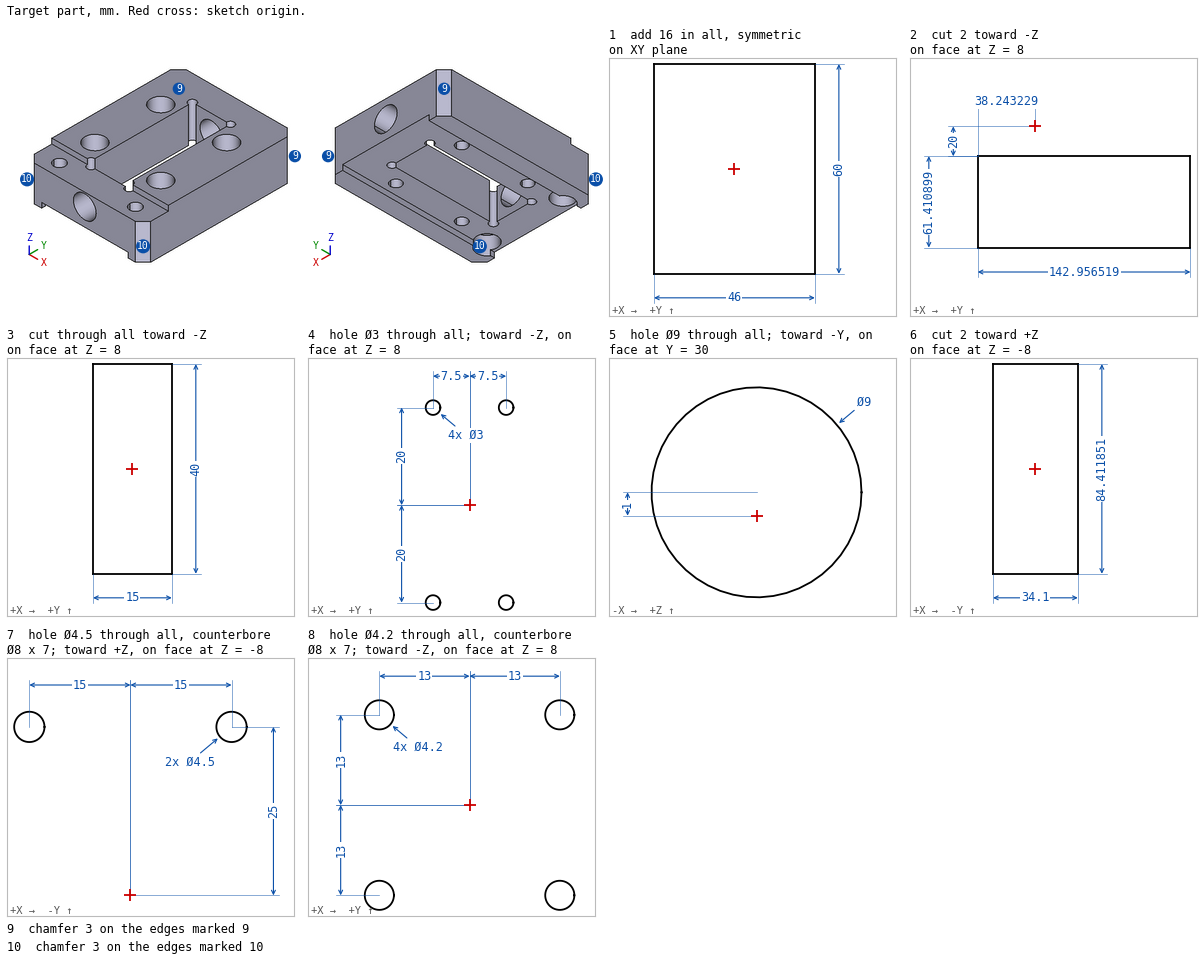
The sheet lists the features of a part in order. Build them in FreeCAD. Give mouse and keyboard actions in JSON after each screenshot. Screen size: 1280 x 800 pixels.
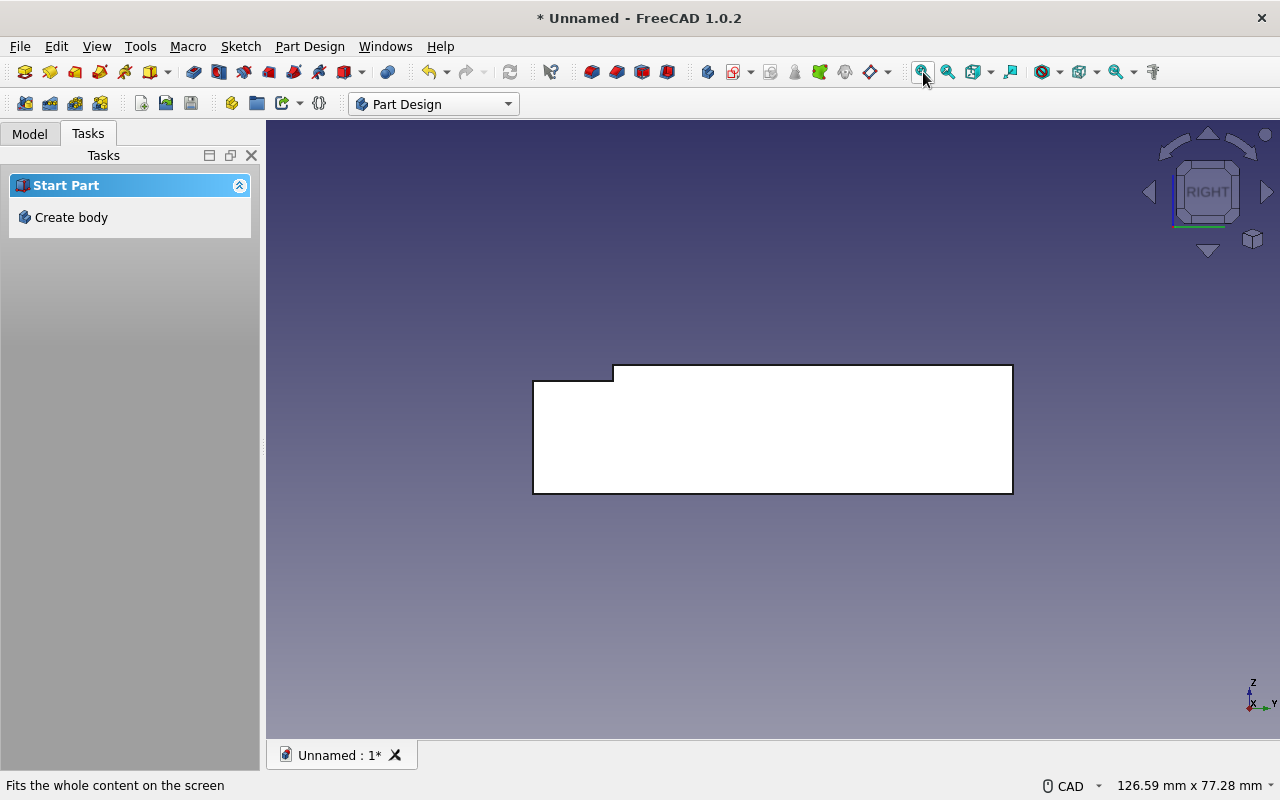
{"action": "left_click", "coordinate": [1013, 428]}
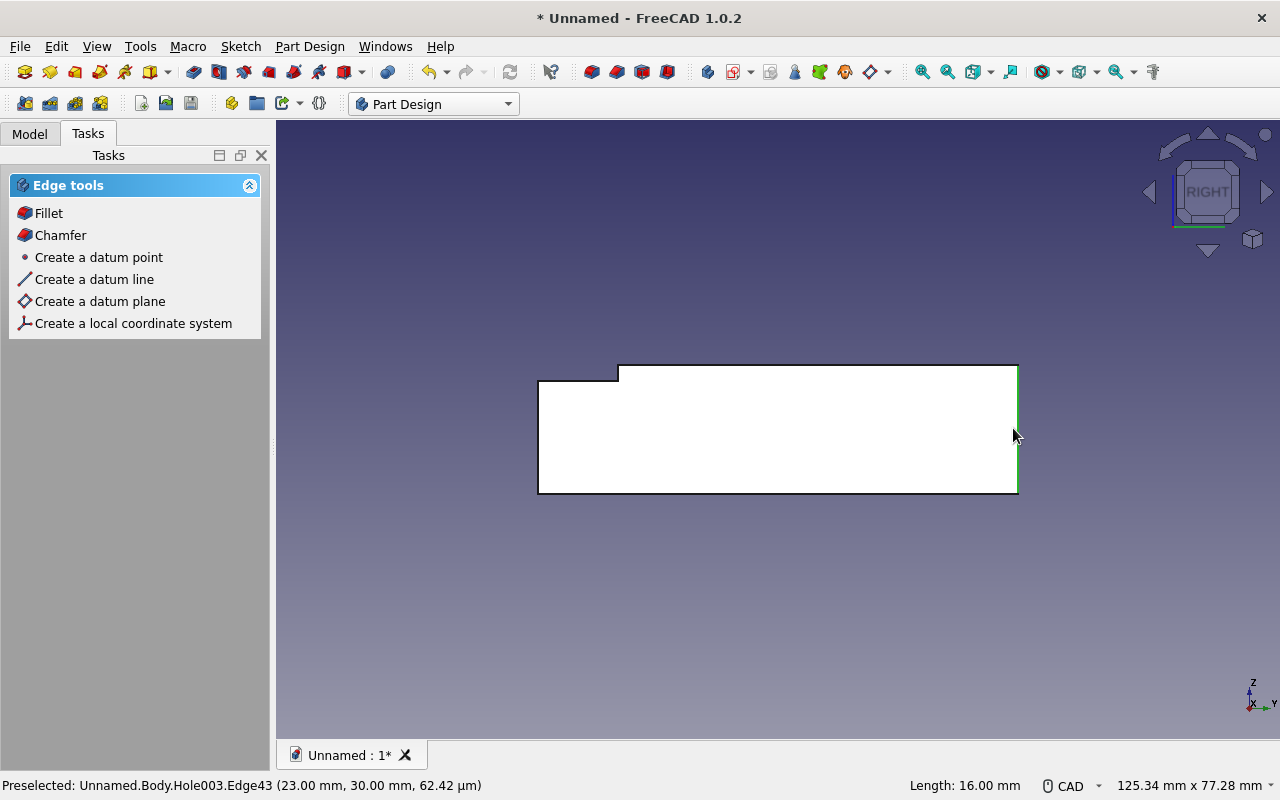
{"action": "key", "text": "5"}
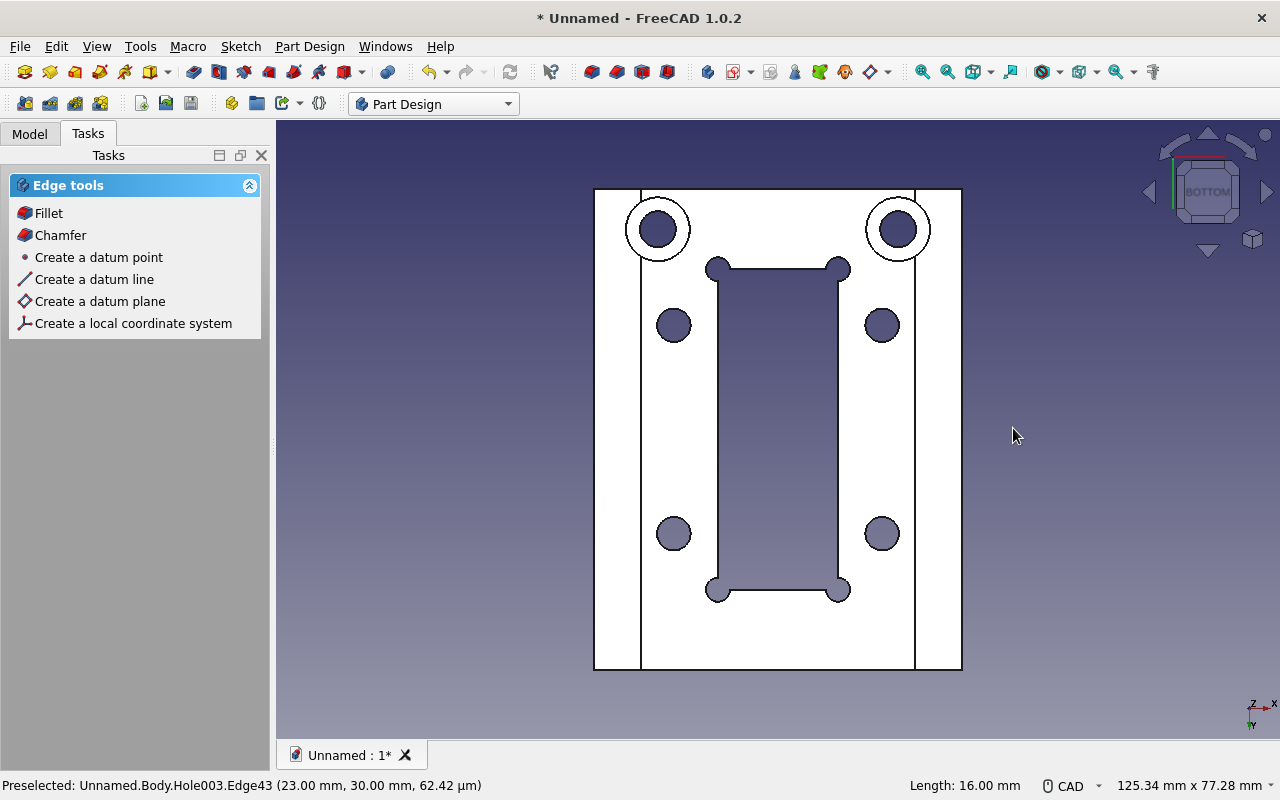
{"action": "key", "text": "4"}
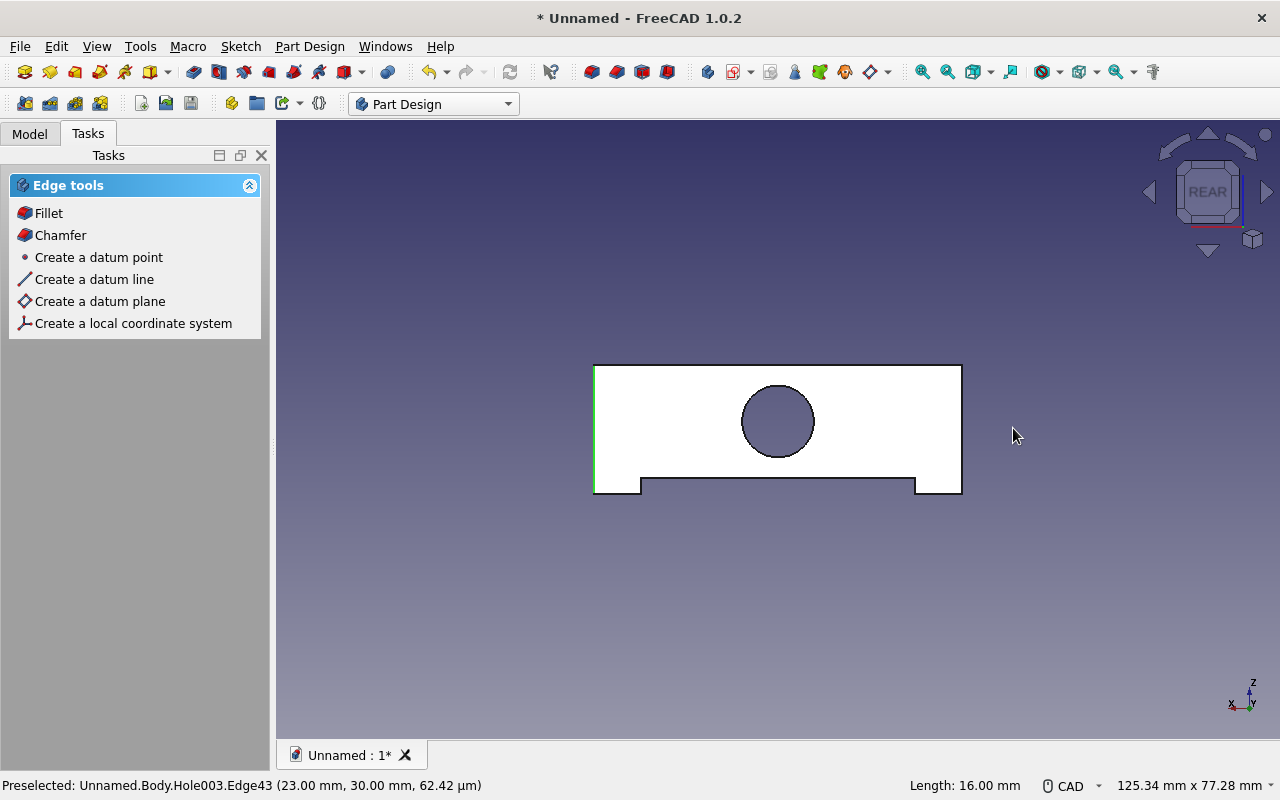
{"action": "left_click", "coordinate": [923, 72]}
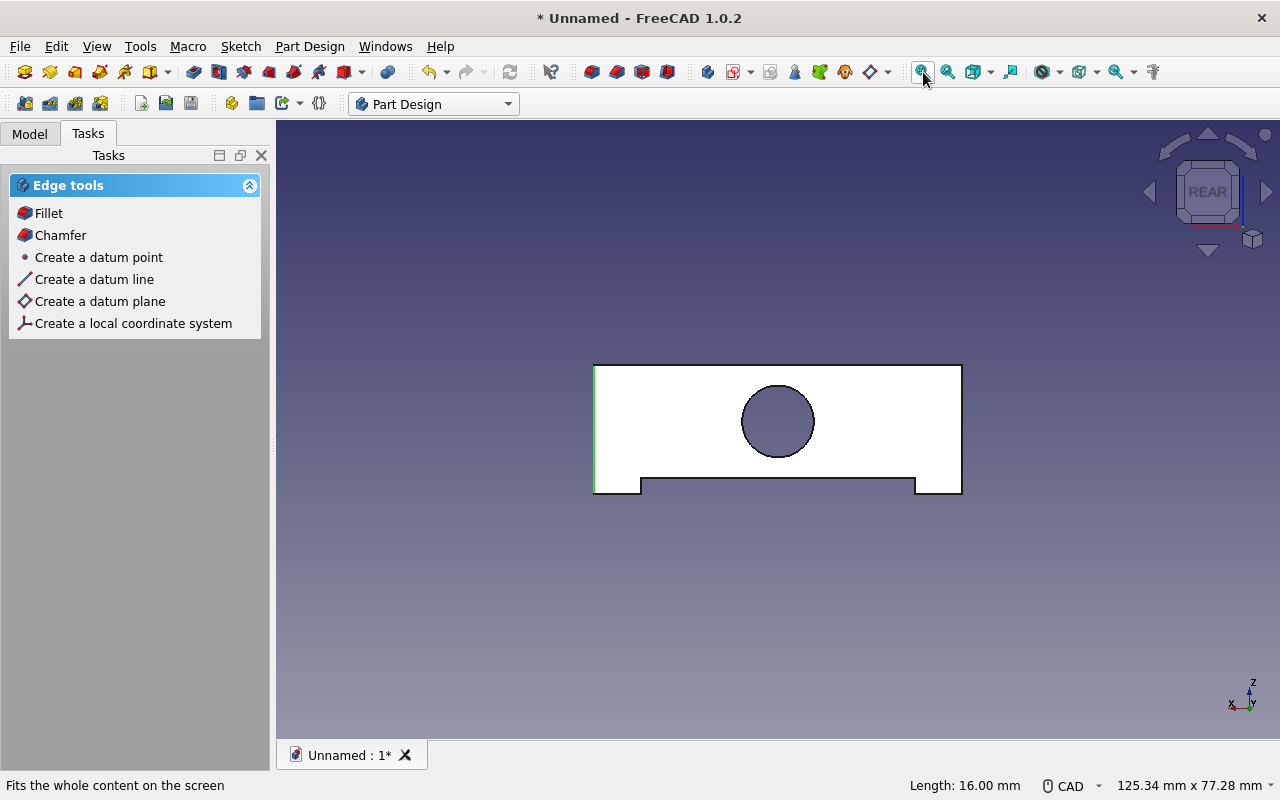
{"action": "left_click", "coordinate": [962, 429], "text": "ctrl"}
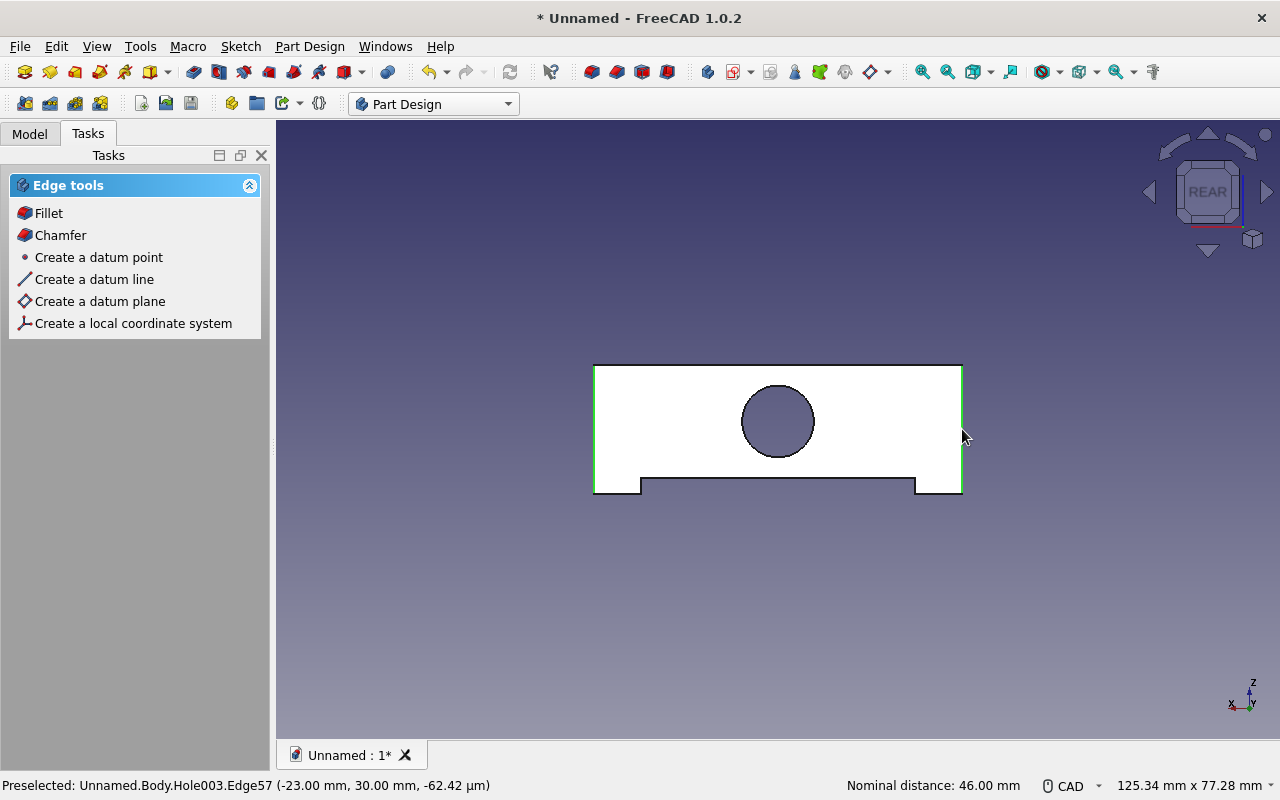
{"action": "left_click", "coordinate": [617, 72]}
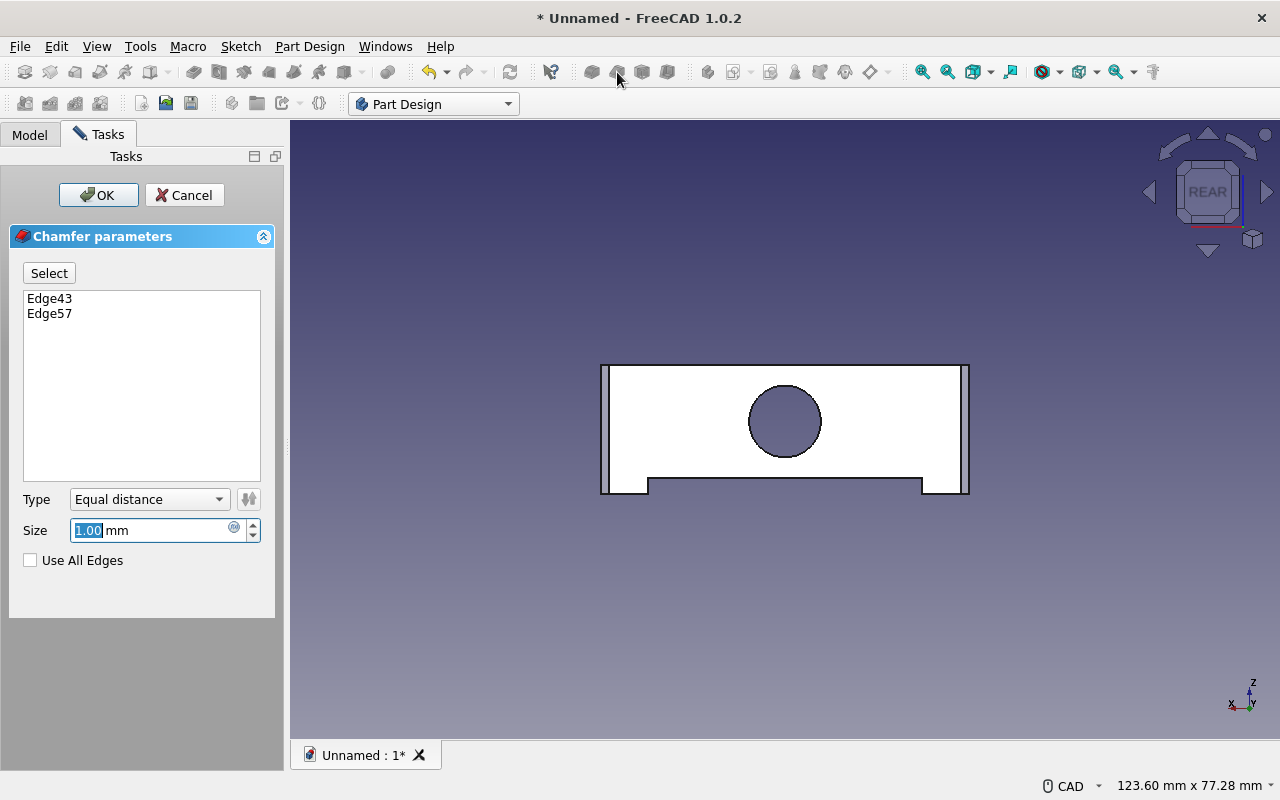
{"action": "type", "text": "3"}
{"action": "key", "text": "Tab"}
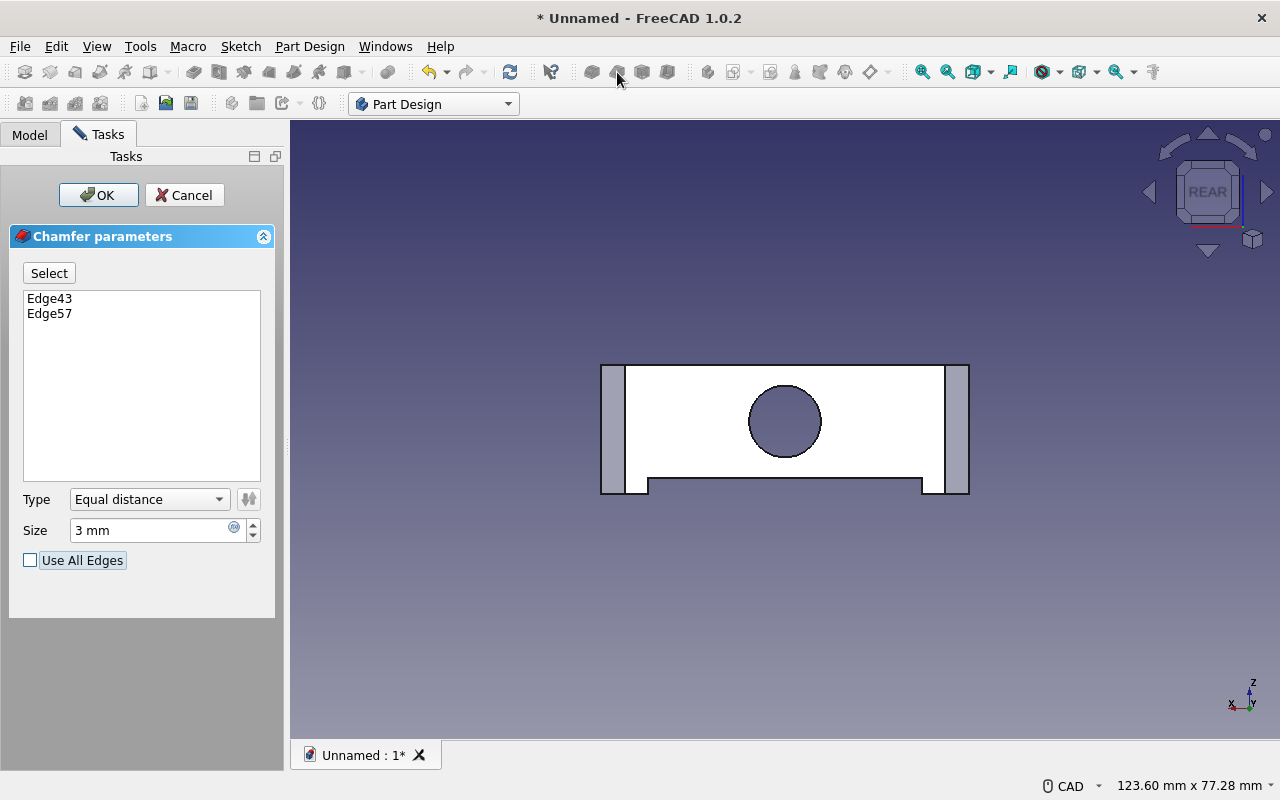
{"action": "left_click", "coordinate": [99, 195]}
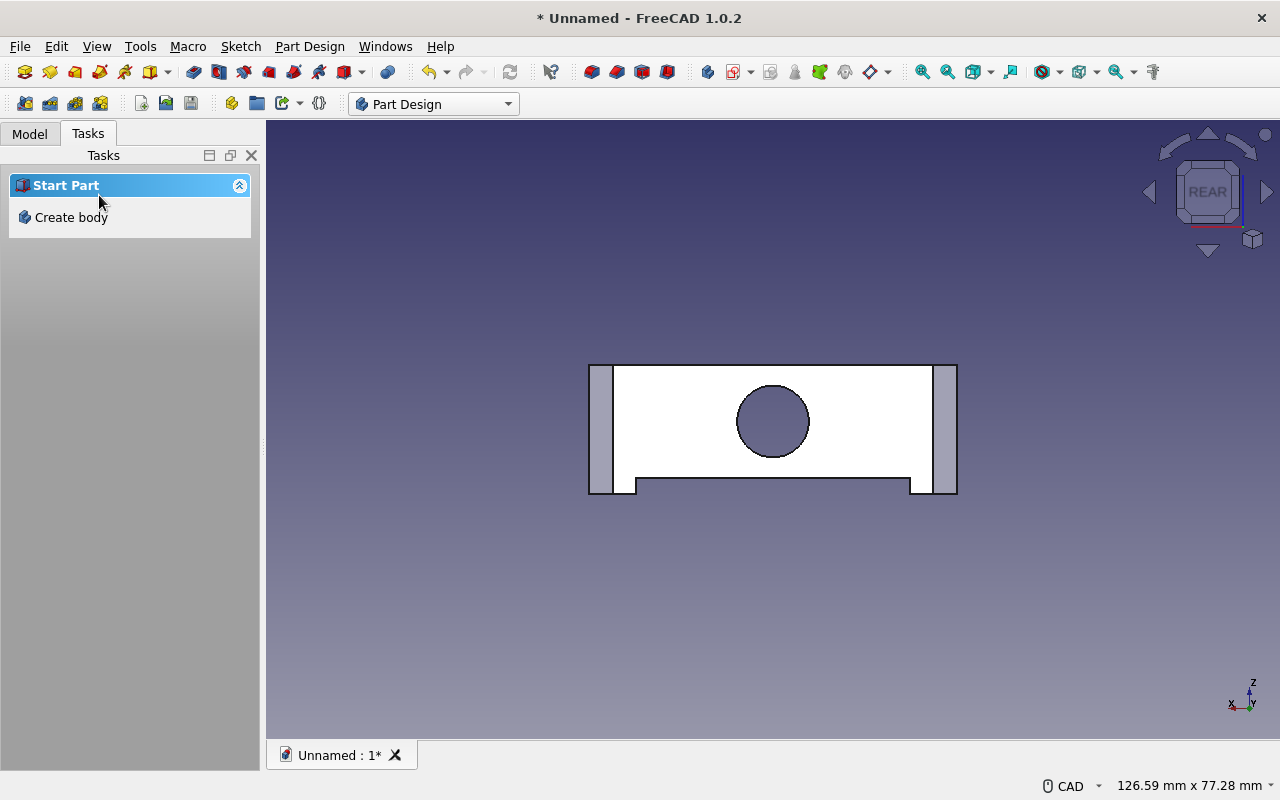
{"action": "left_click", "coordinate": [923, 72]}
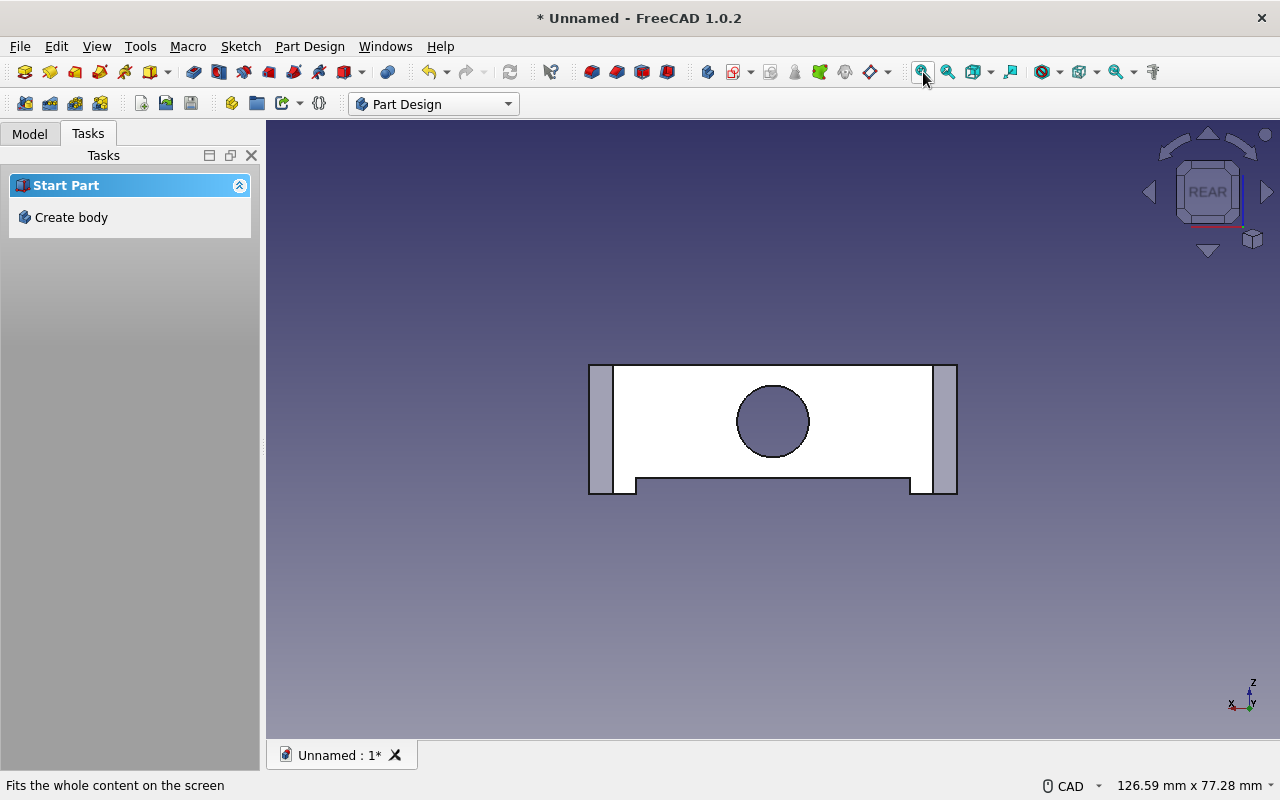
{"action": "key", "text": "0"}